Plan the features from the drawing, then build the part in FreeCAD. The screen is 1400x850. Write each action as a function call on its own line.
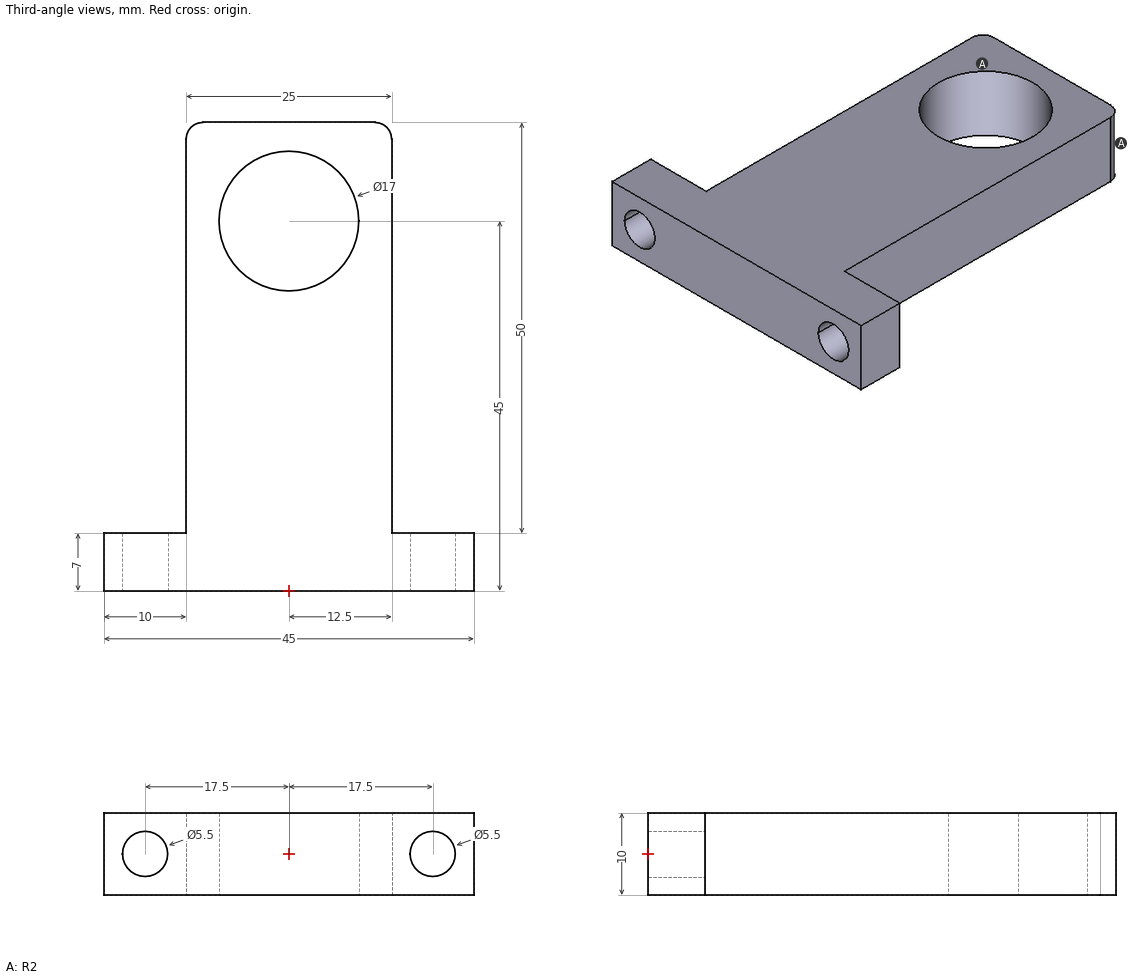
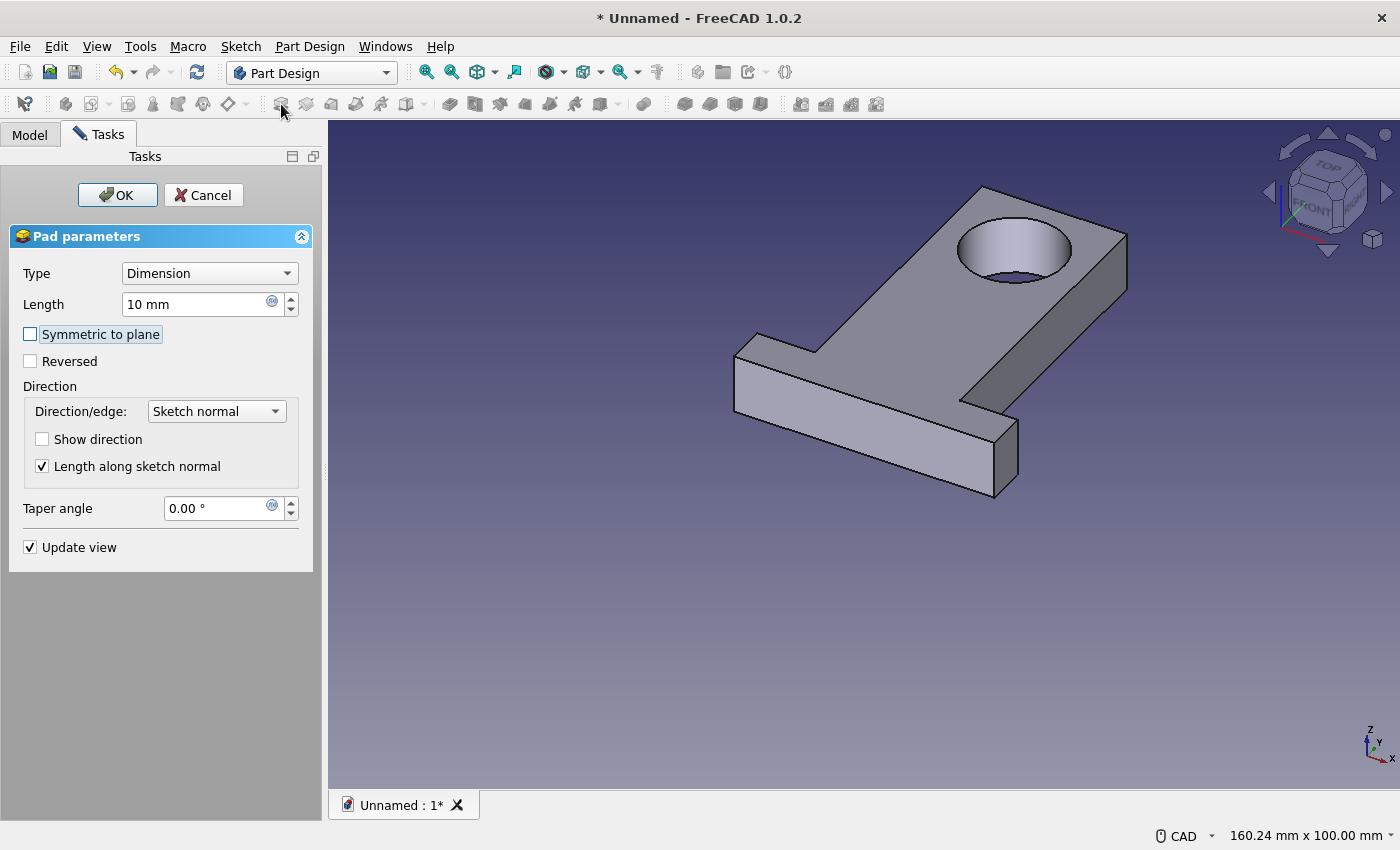
click(31, 334)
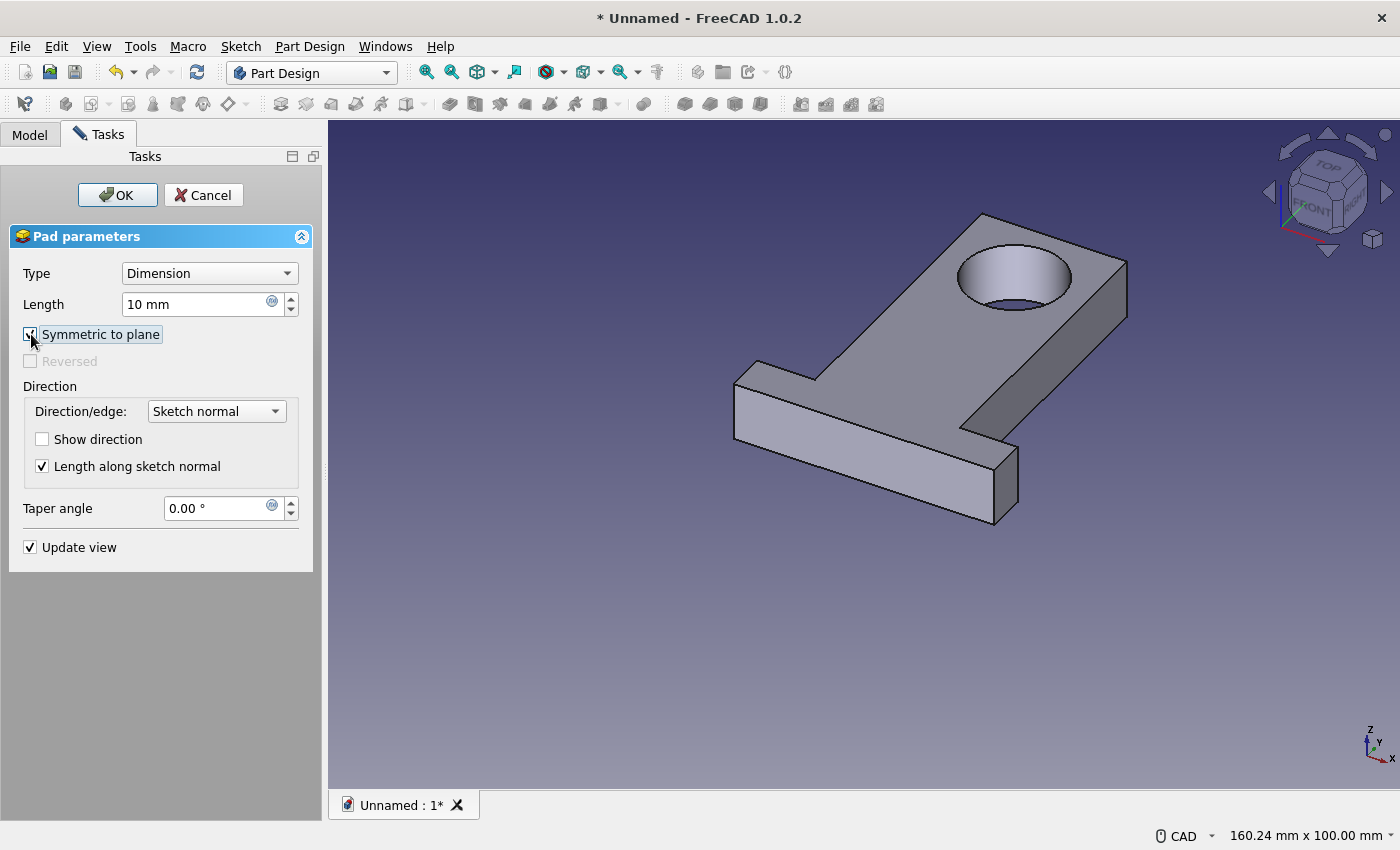
click(118, 195)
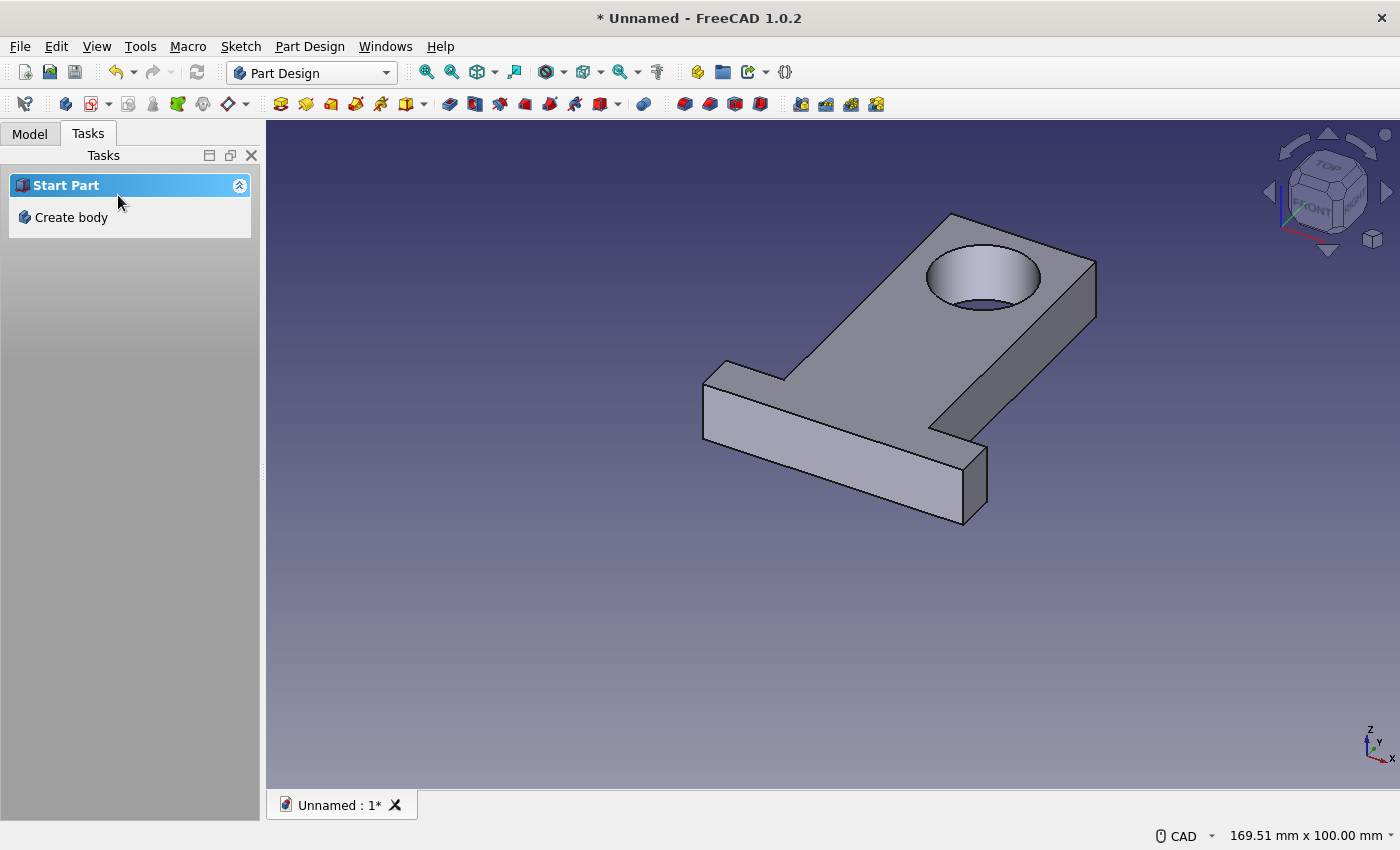
key(0)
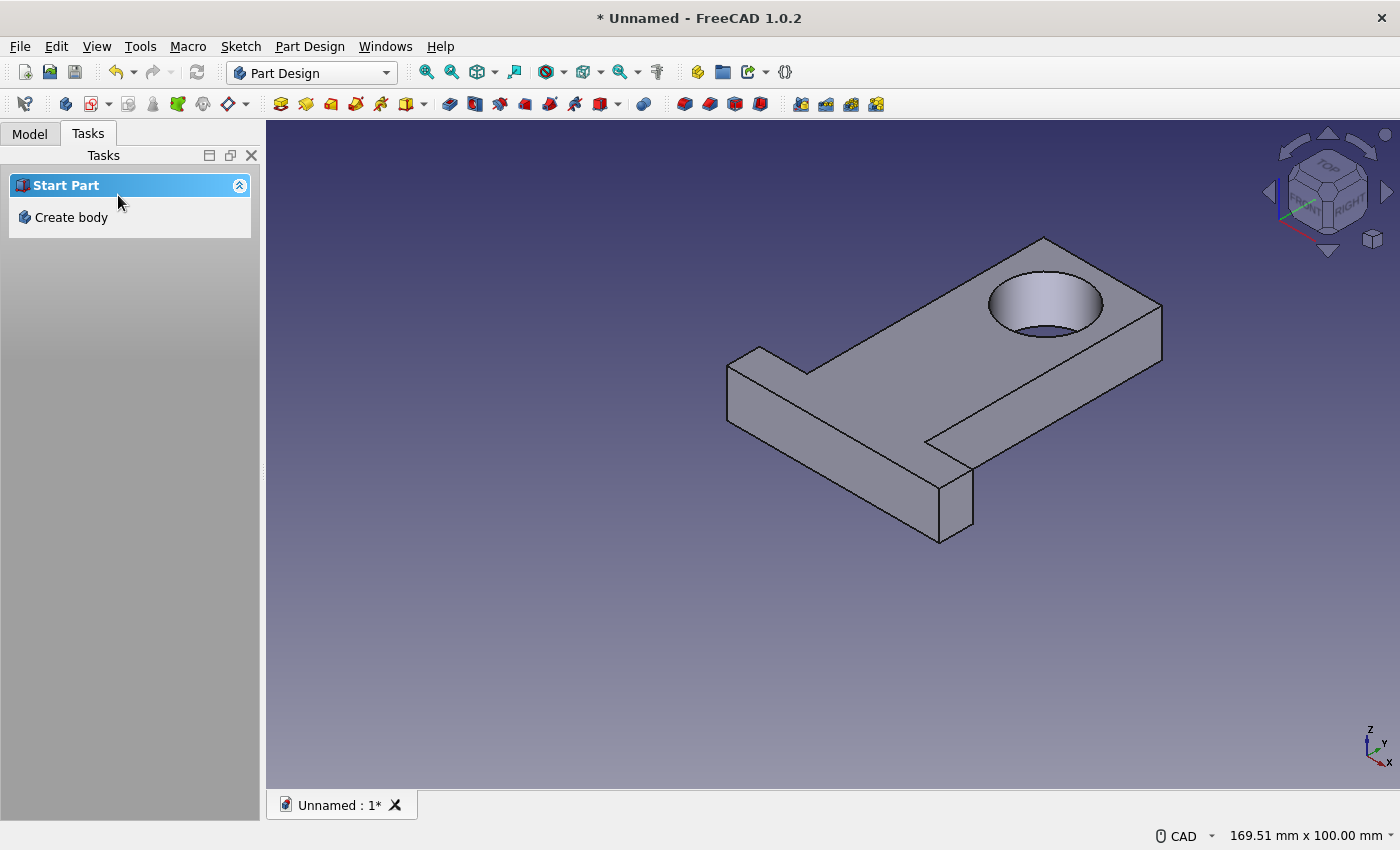
key(2)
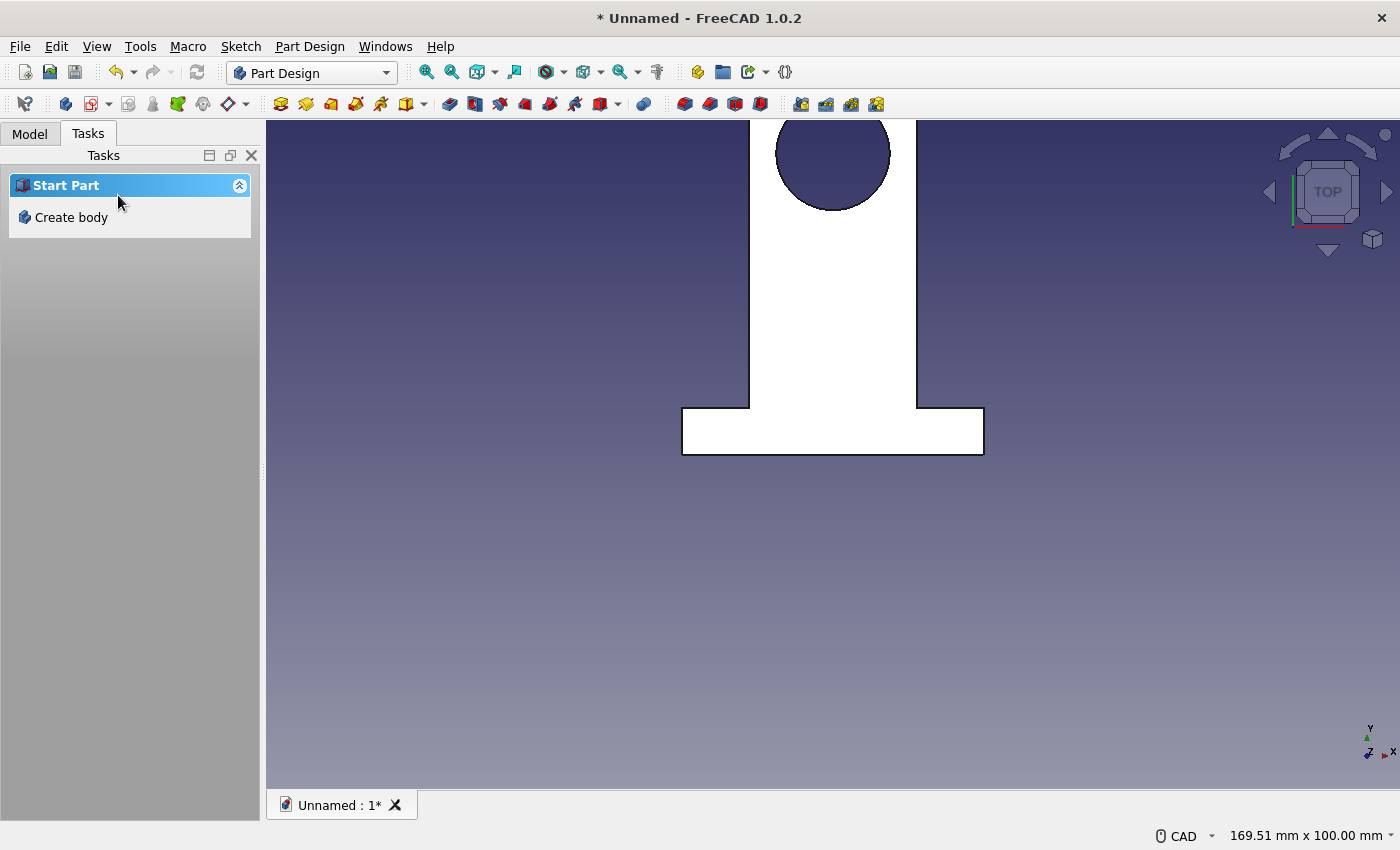
key(v)
key(f)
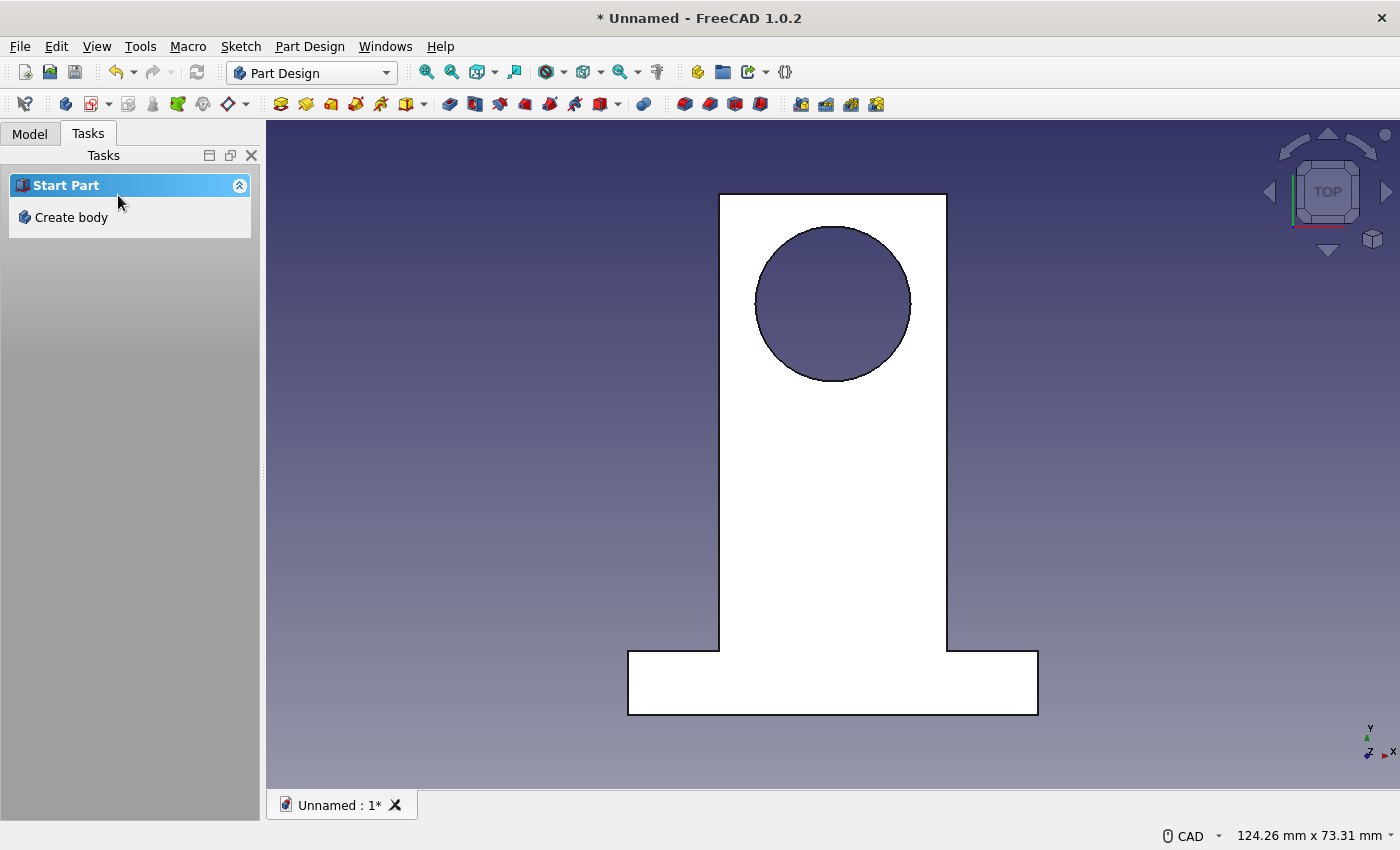
key(1)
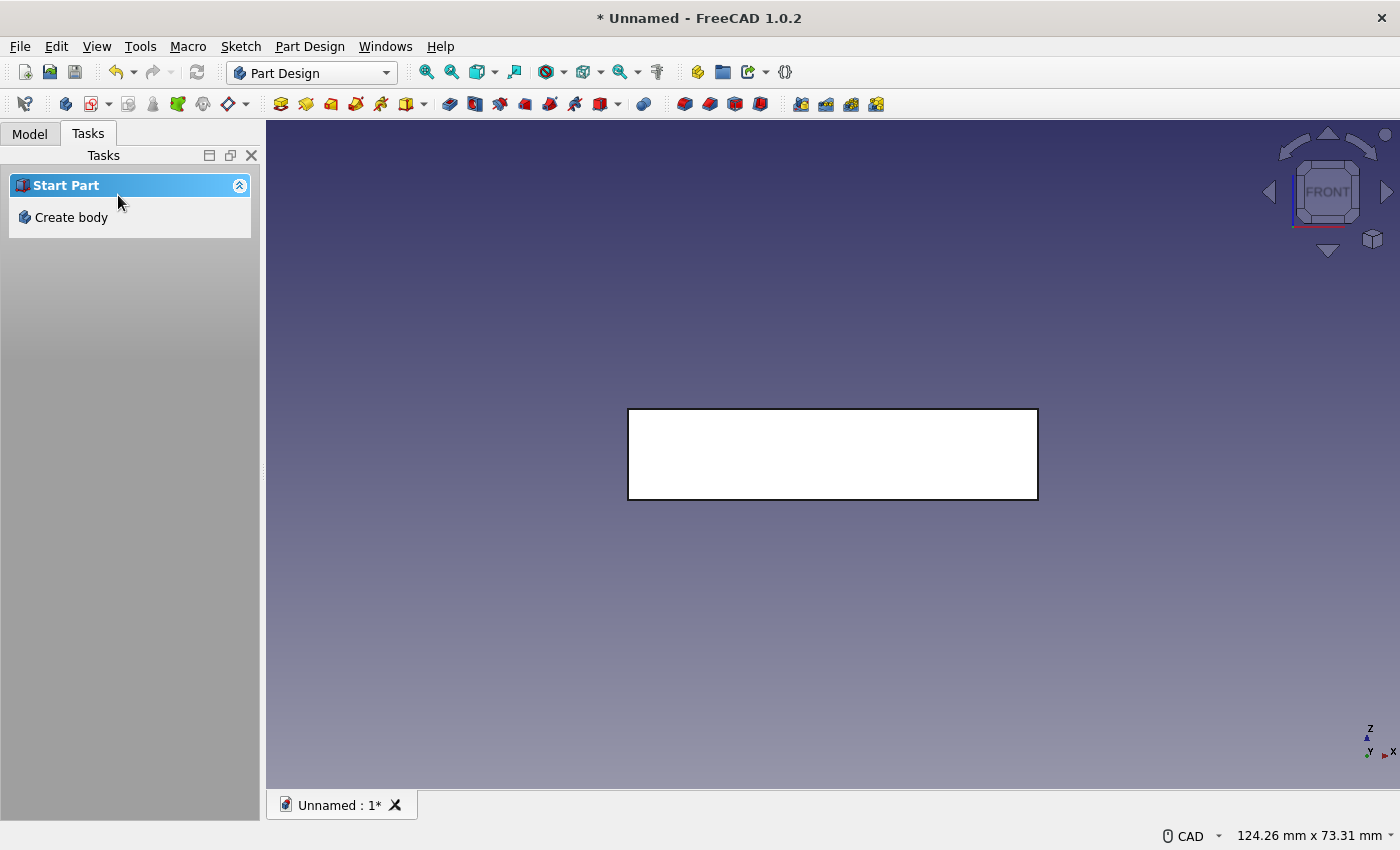
click(427, 72)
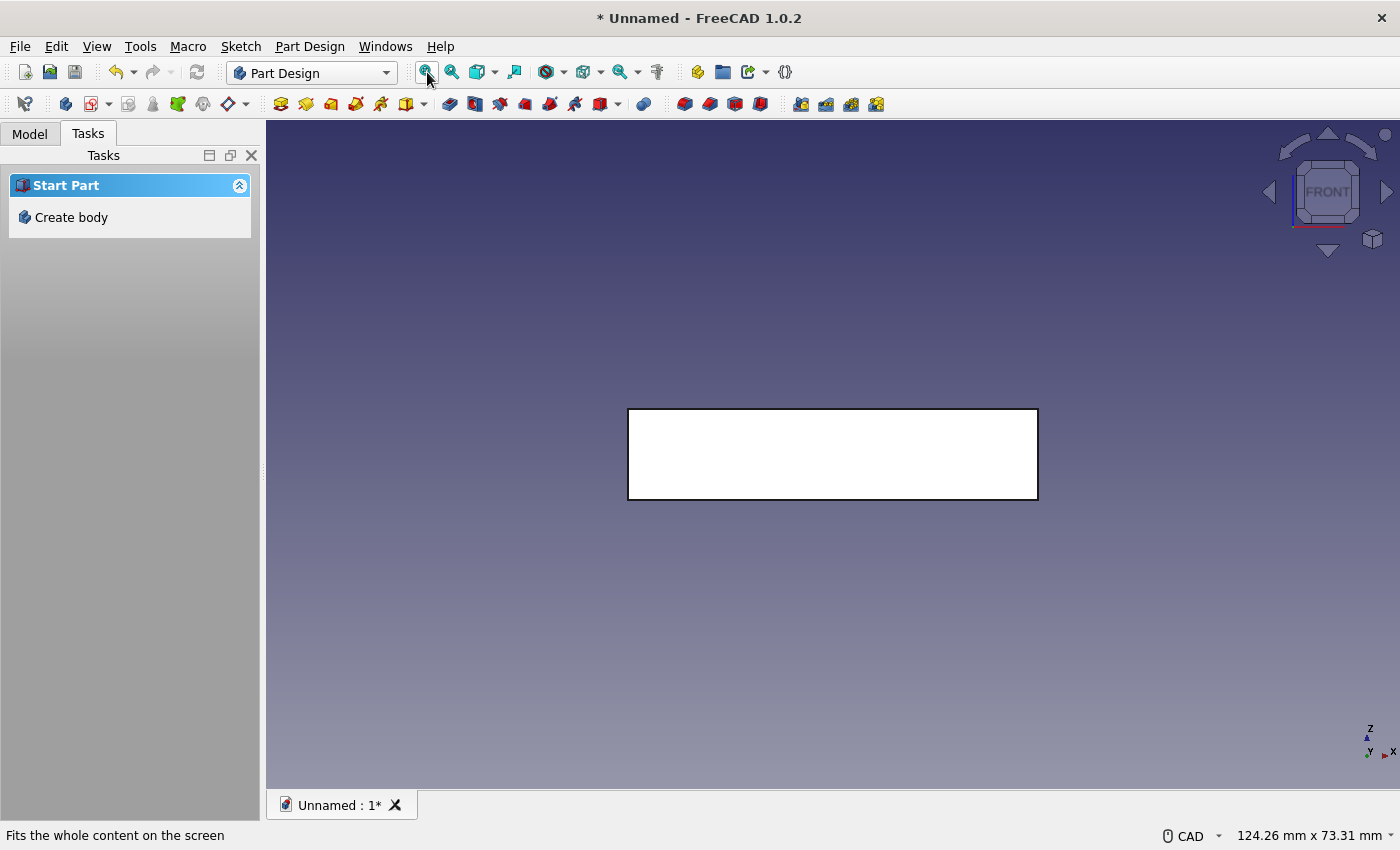
key(3)